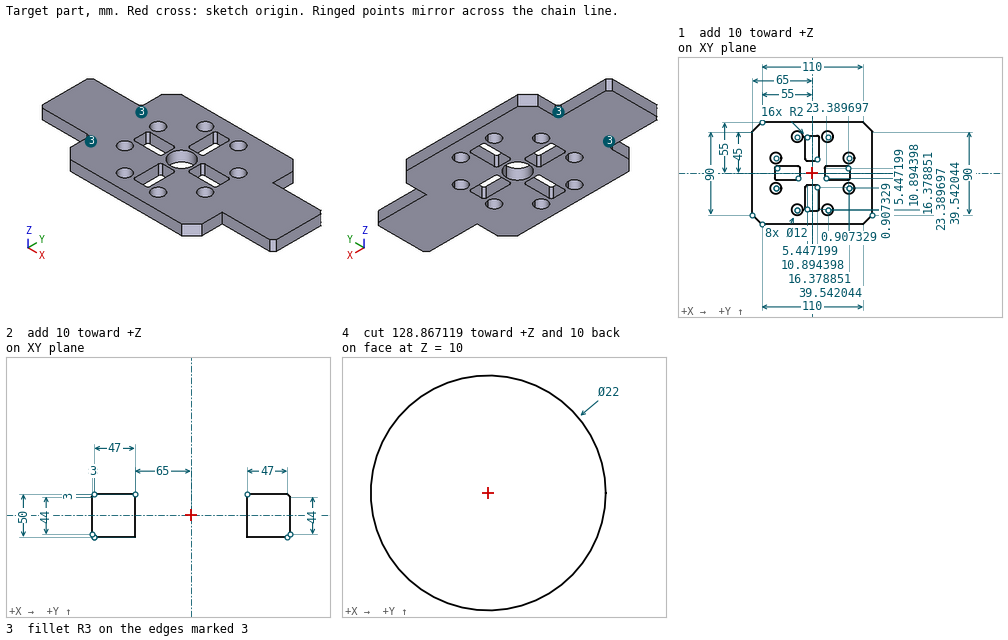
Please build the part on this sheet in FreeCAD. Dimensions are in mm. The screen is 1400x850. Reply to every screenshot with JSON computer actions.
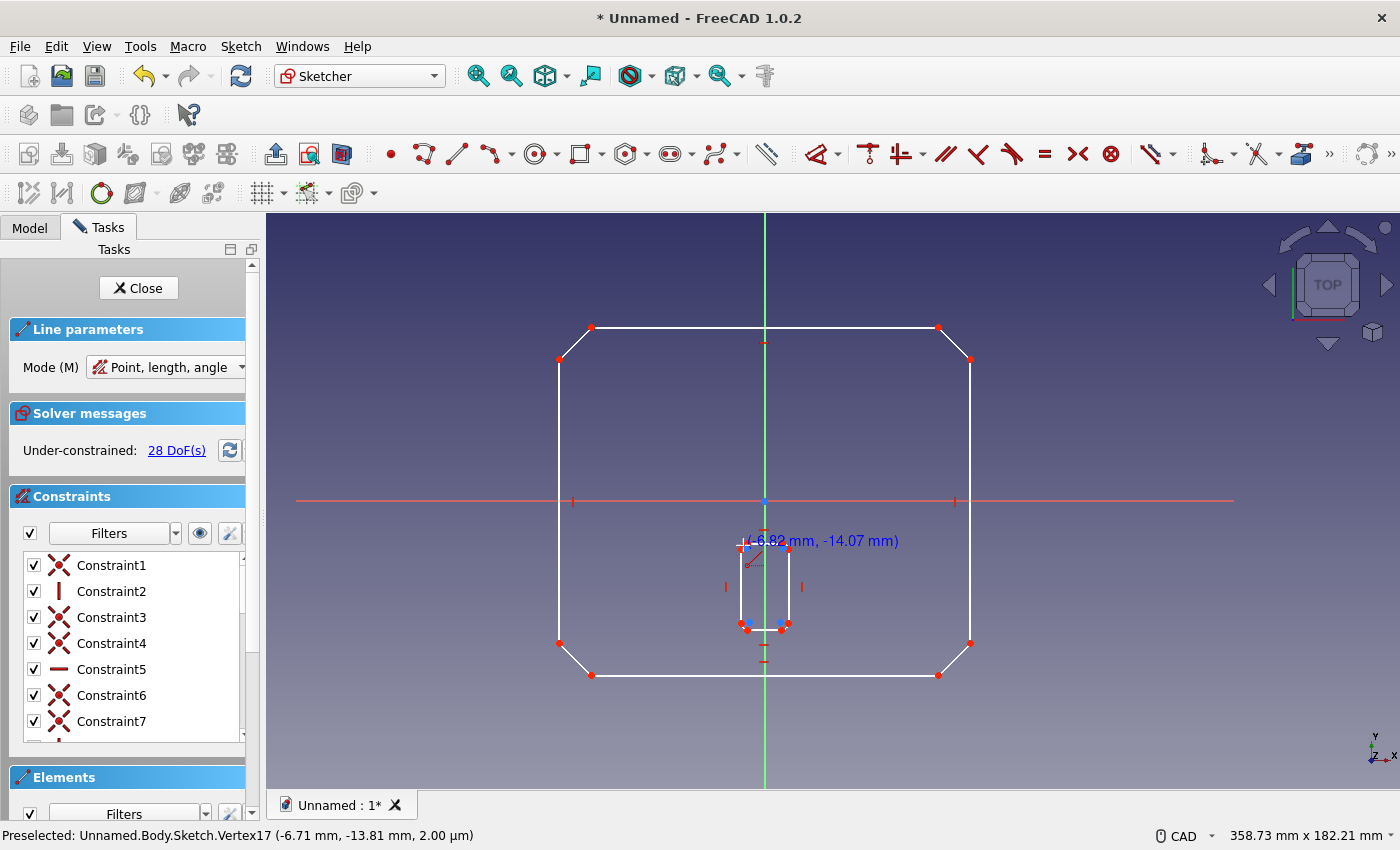
{"action": "left_click", "coordinate": [807, 518]}
{"action": "left_click", "coordinate": [807, 484]}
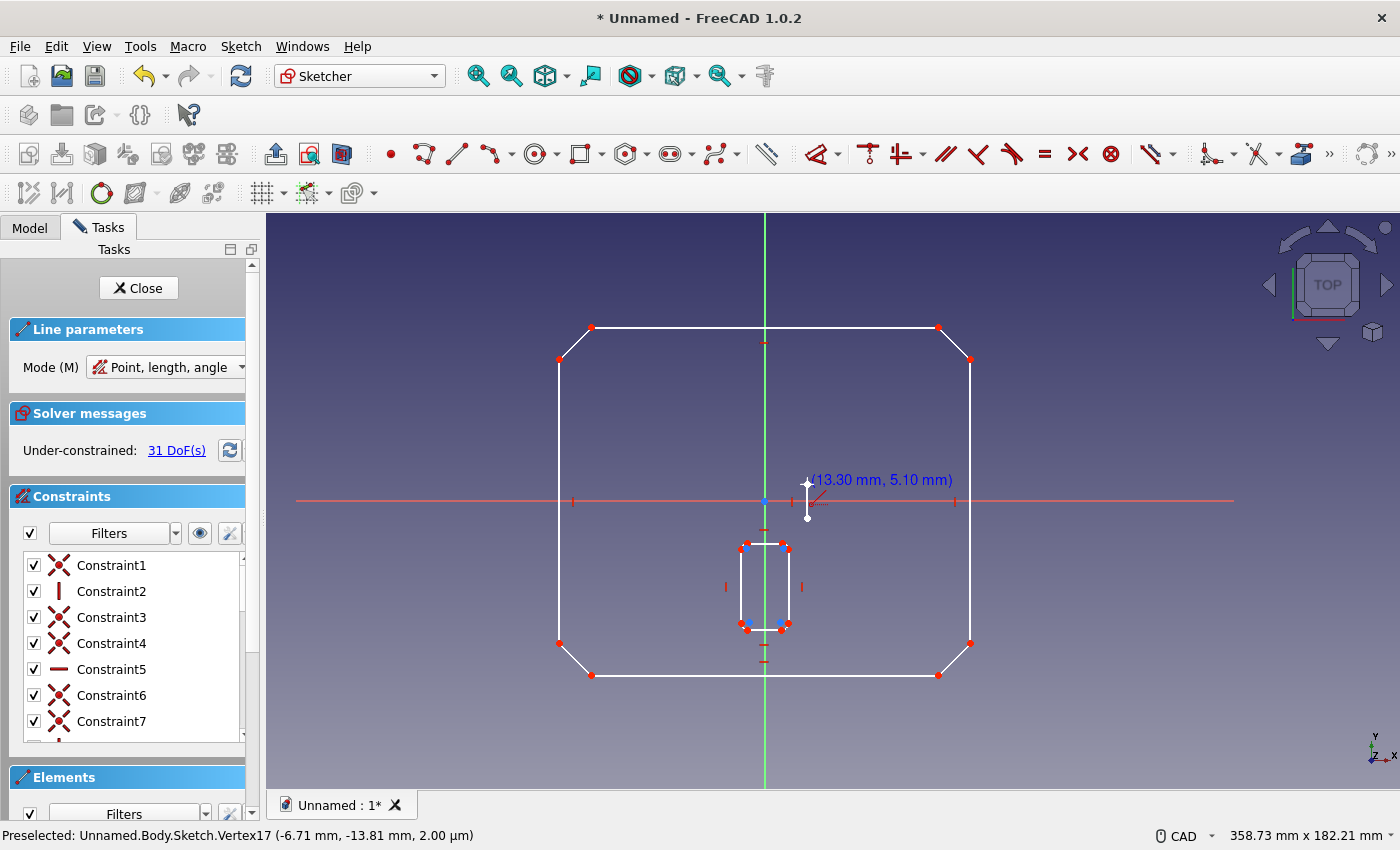
{"action": "scroll", "coordinate": [813, 478], "scroll_direction": "up", "scroll_amount": 3}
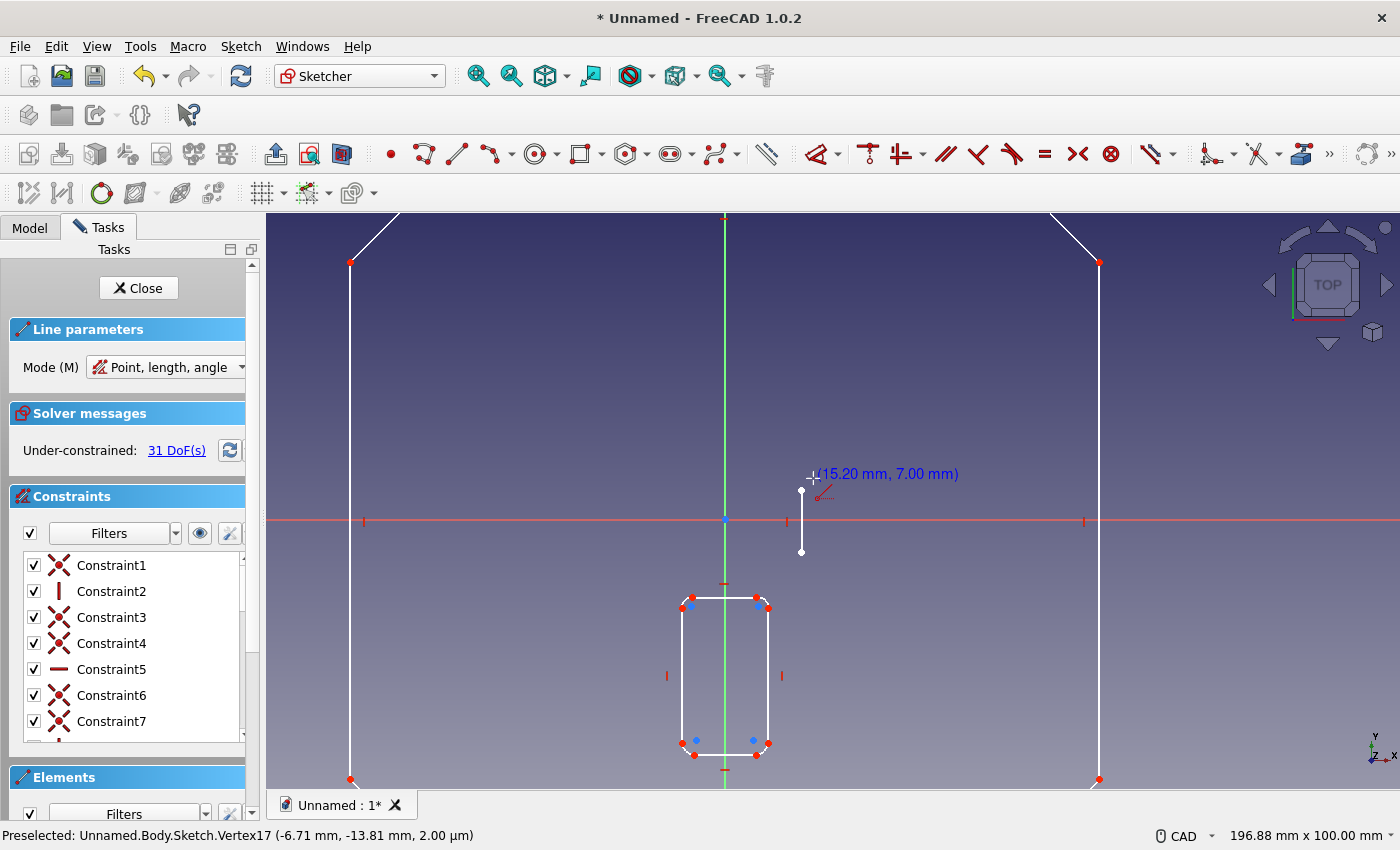
{"action": "left_click", "coordinate": [813, 477]}
{"action": "left_click", "coordinate": [948, 477]}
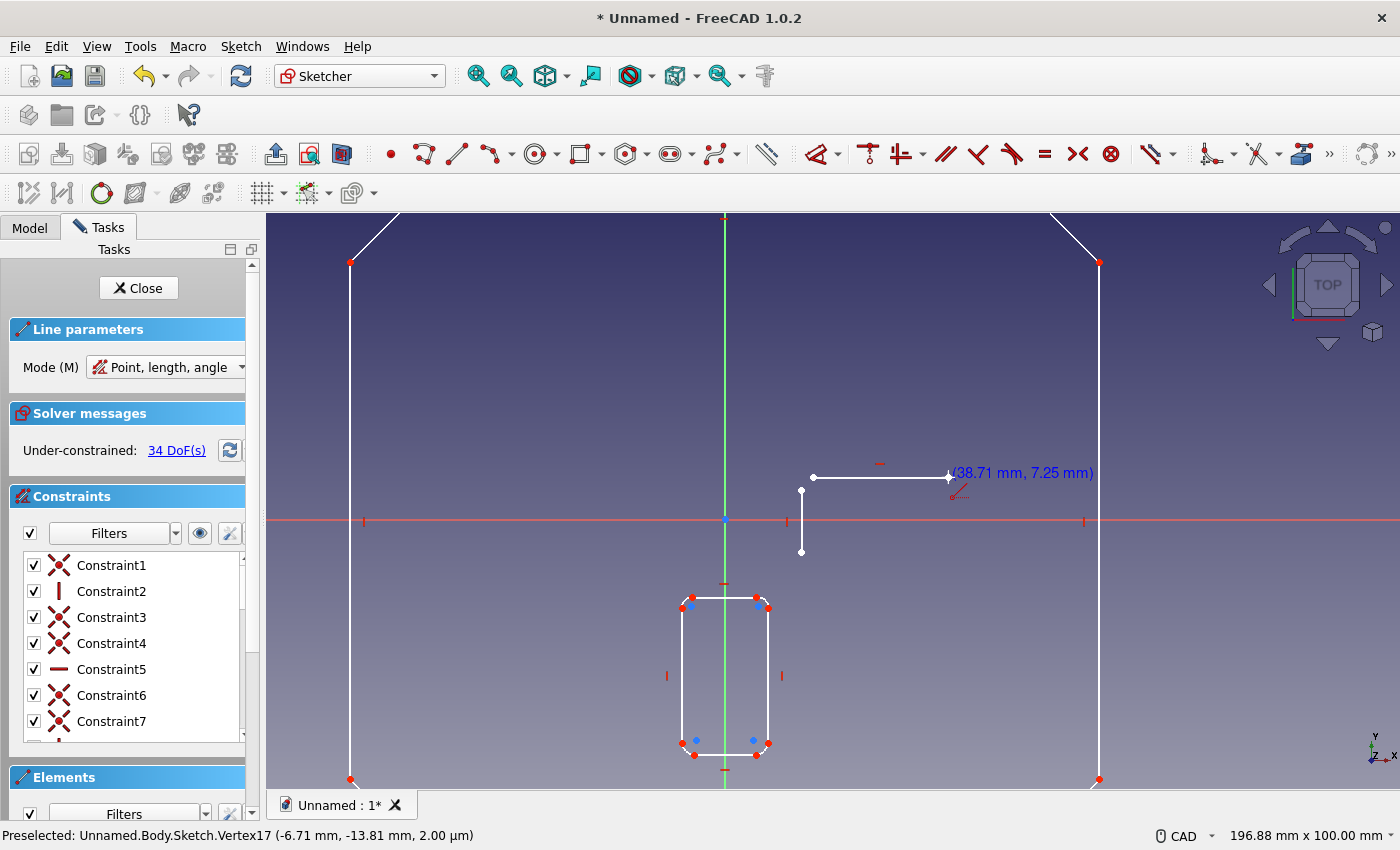
{"action": "left_click", "coordinate": [959, 488]}
{"action": "left_click", "coordinate": [959, 551]}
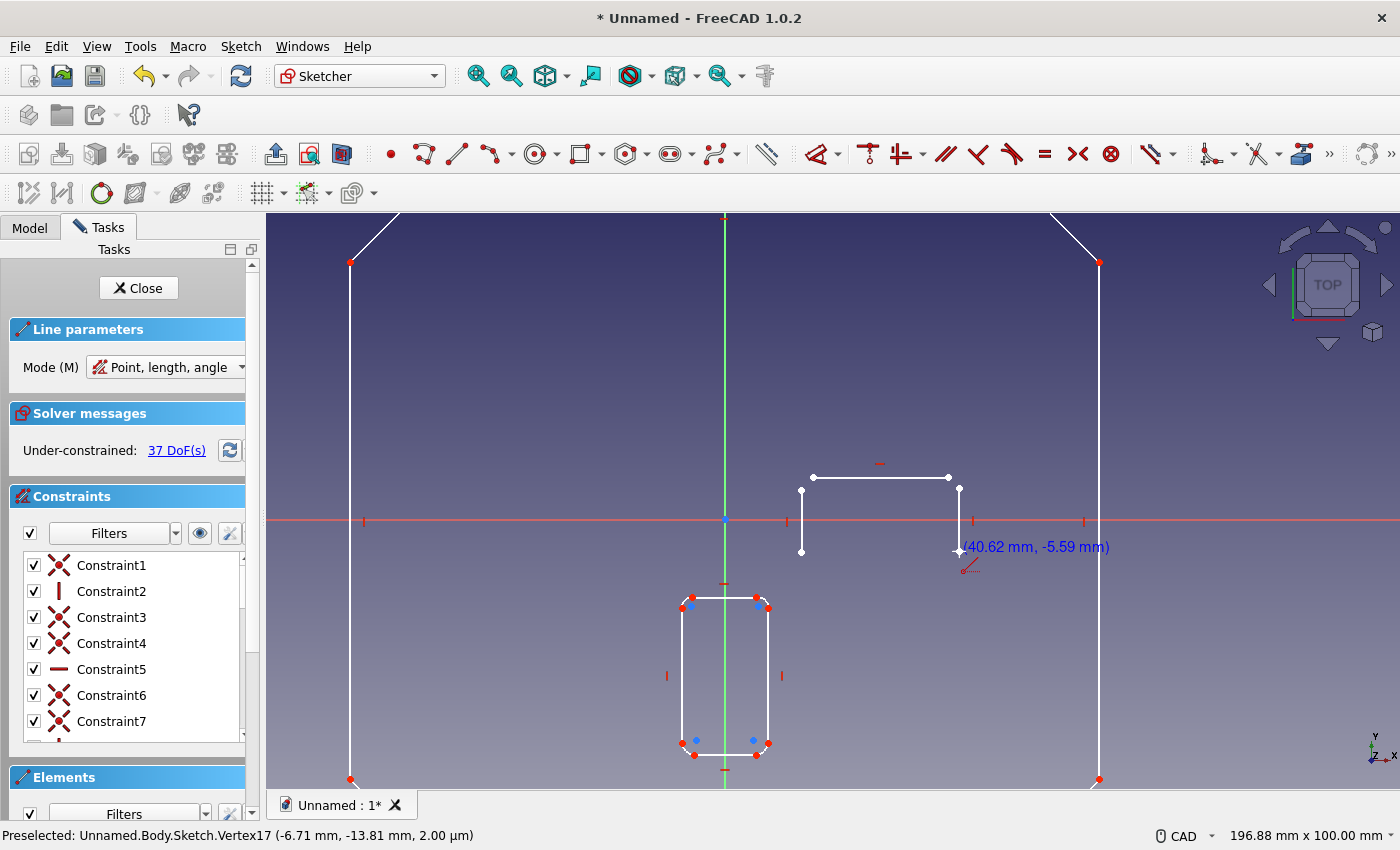
{"action": "left_click", "coordinate": [948, 563]}
{"action": "left_click", "coordinate": [813, 563]}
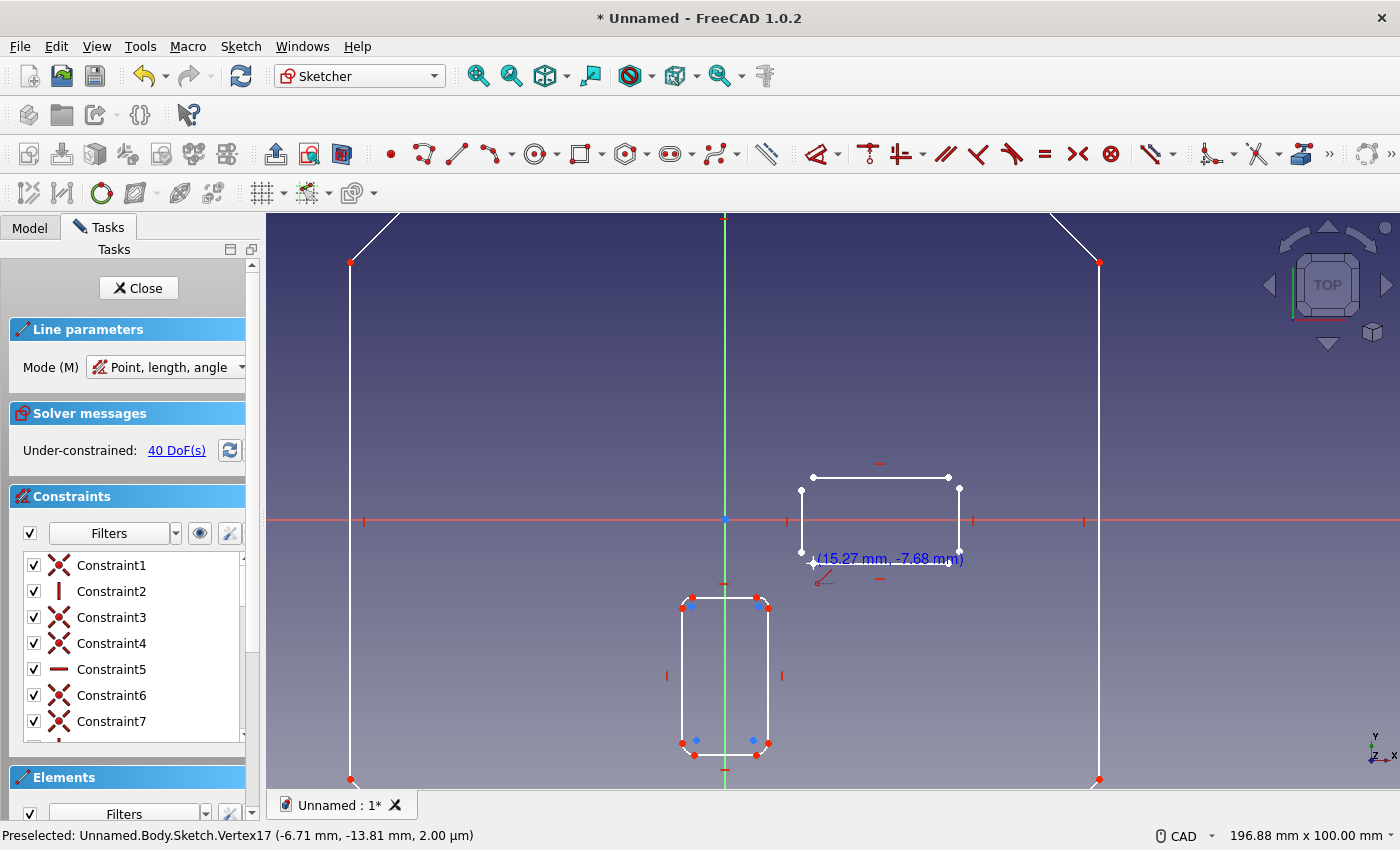
{"action": "left_click", "coordinate": [490, 154]}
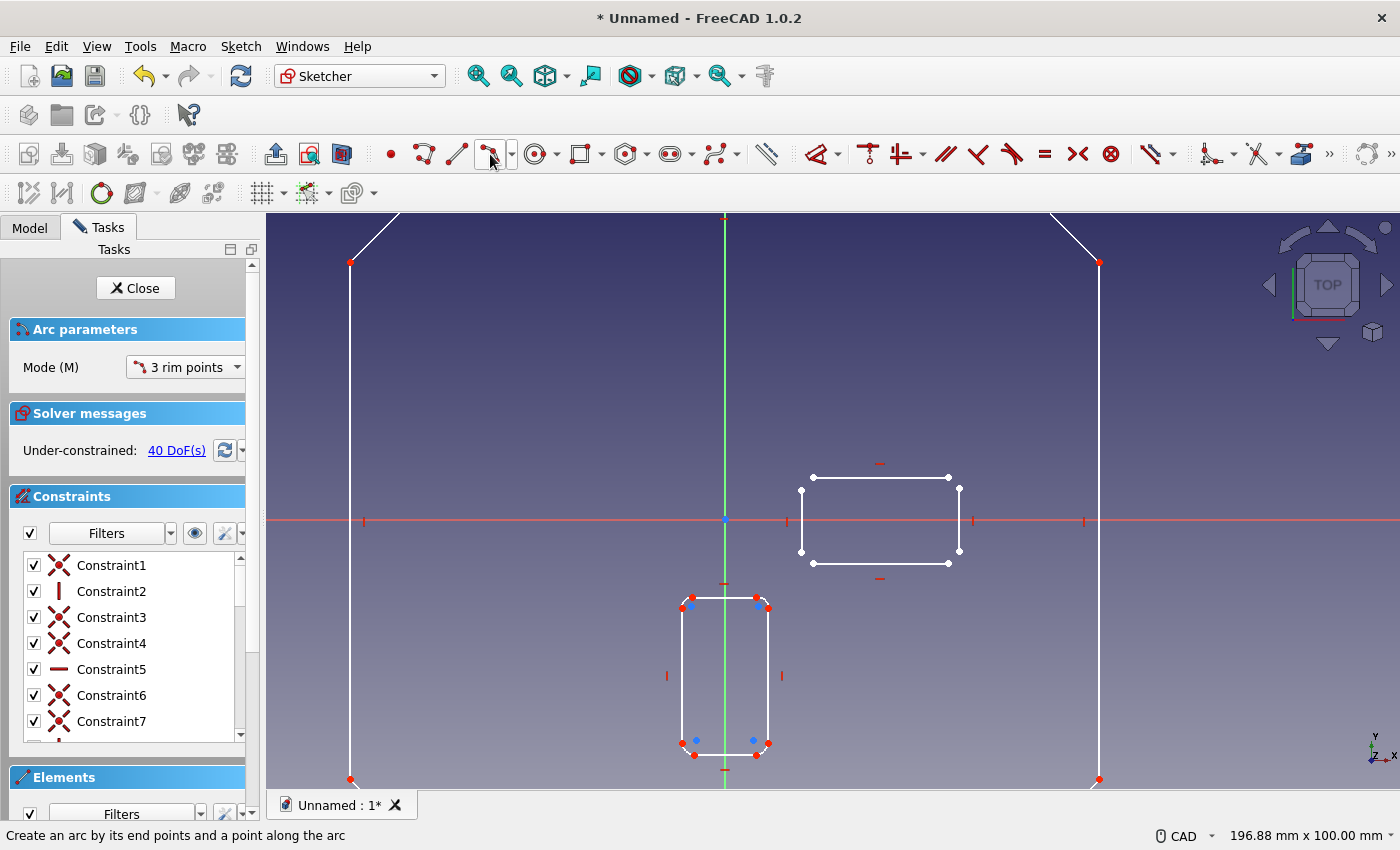
{"action": "left_click", "coordinate": [802, 490]}
{"action": "left_click", "coordinate": [813, 478]}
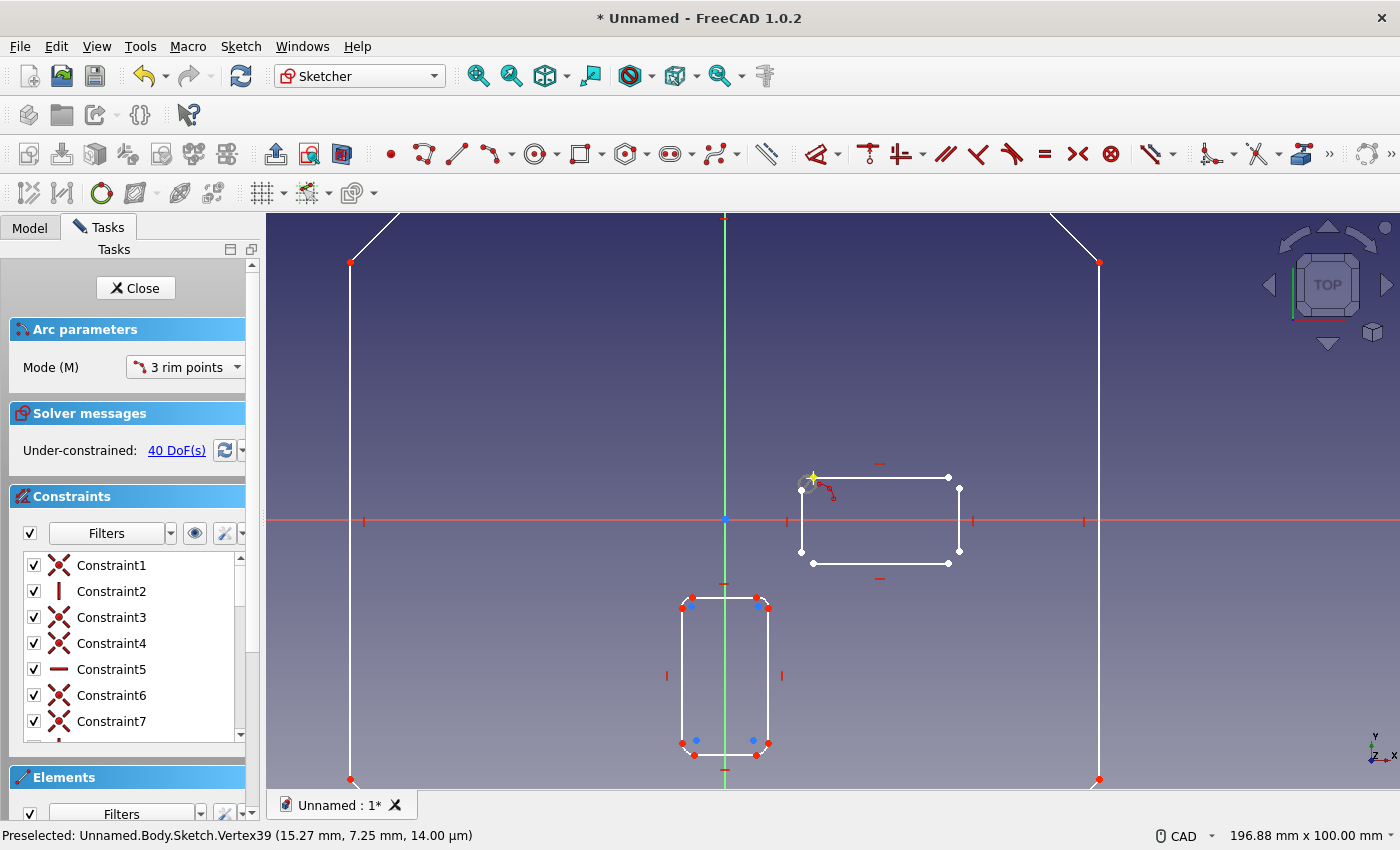
{"action": "scroll", "coordinate": [805, 480], "scroll_direction": "up", "scroll_amount": 8}